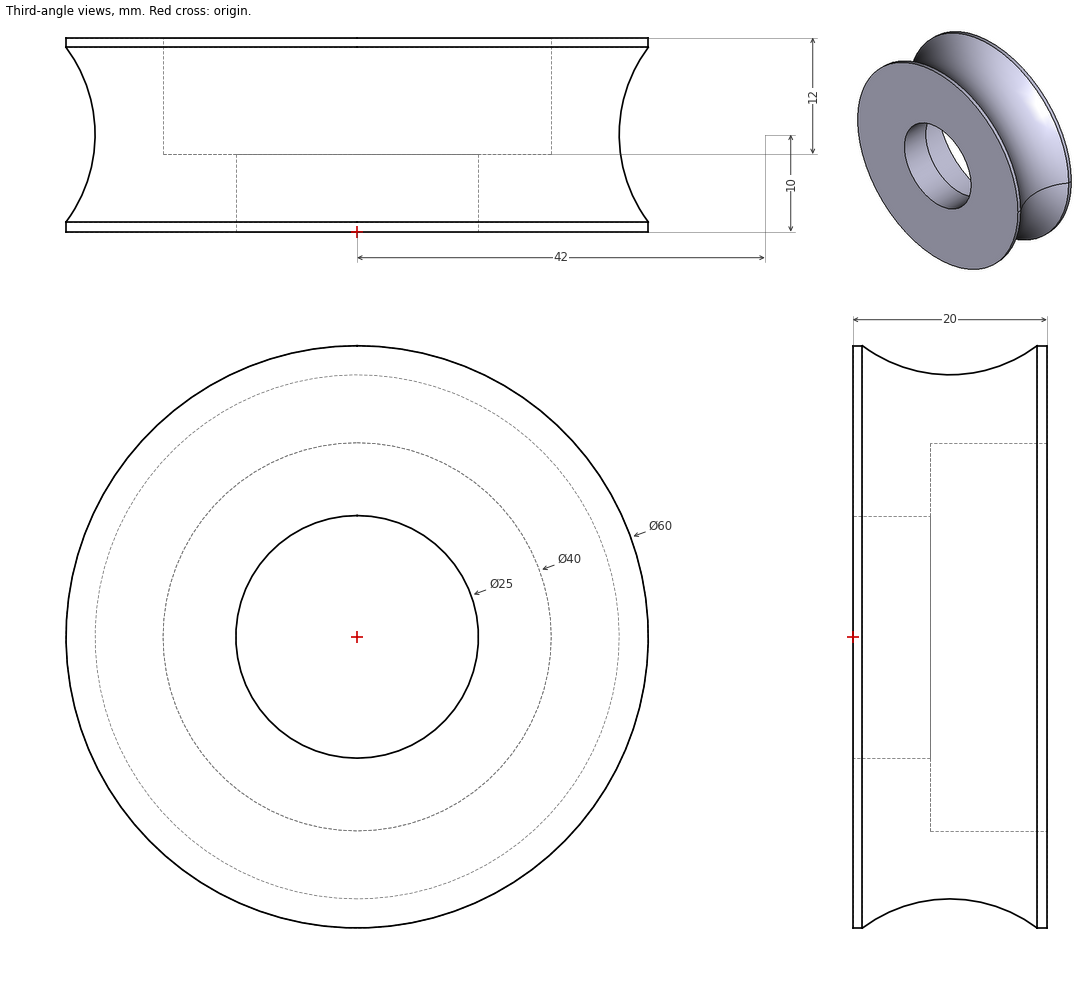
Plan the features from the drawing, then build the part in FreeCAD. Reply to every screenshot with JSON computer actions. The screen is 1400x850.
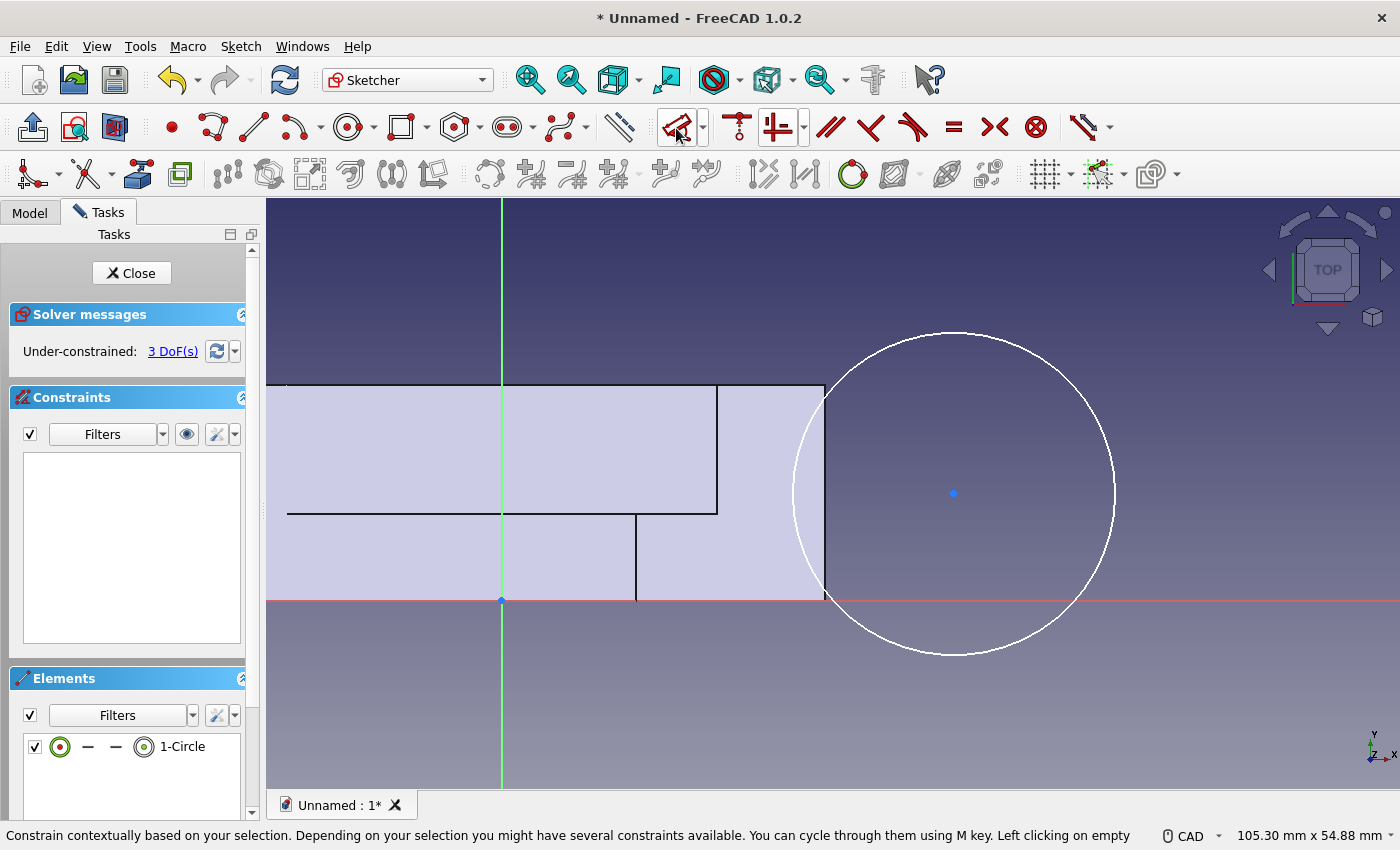
{"action": "left_click", "coordinate": [1068, 380]}
{"action": "left_click", "coordinate": [1091, 357]}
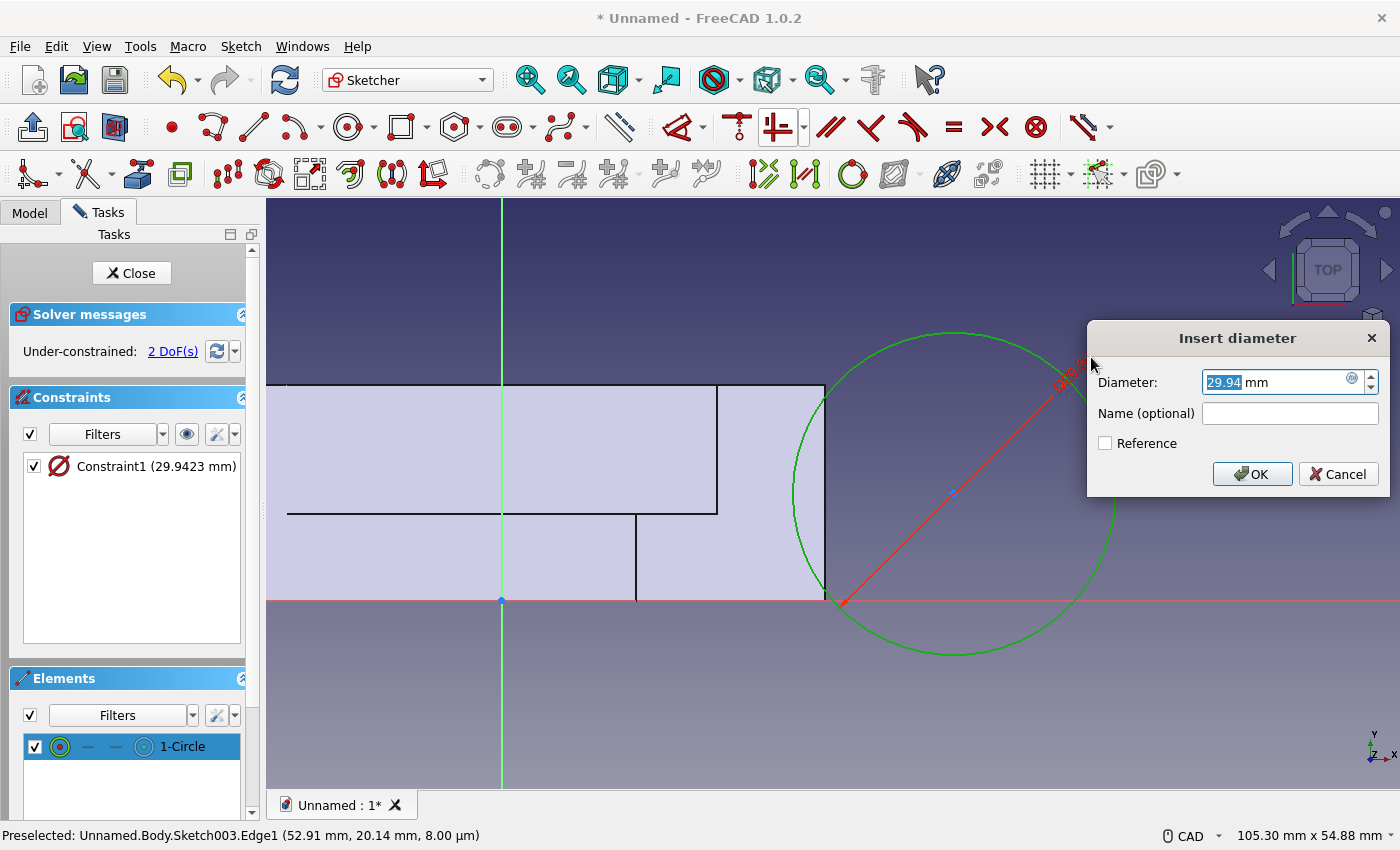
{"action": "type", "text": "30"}
{"action": "key", "text": "Return"}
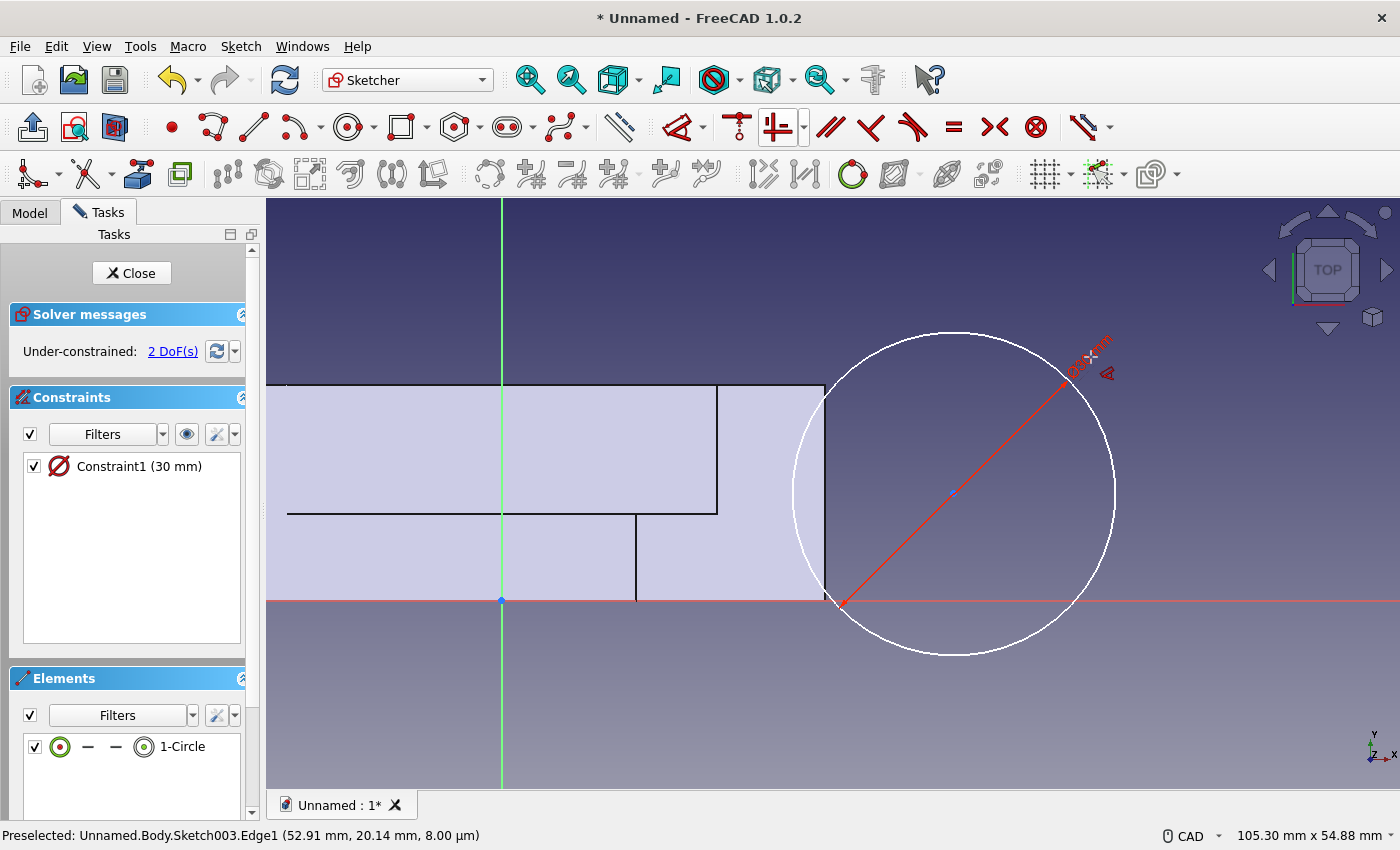
{"action": "left_click", "coordinate": [954, 494]}
{"action": "left_click", "coordinate": [728, 635]}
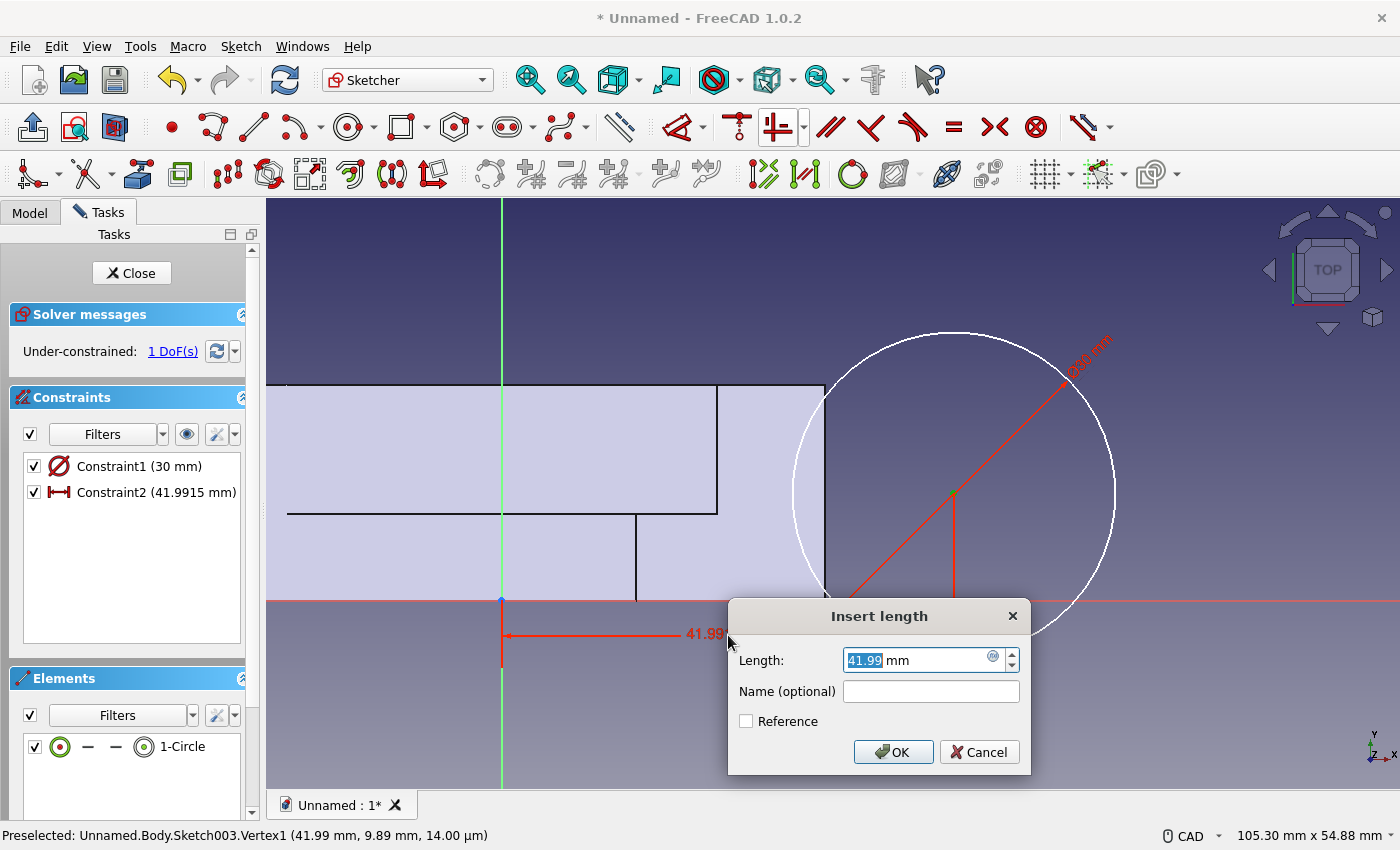
{"action": "type", "text": "42"}
{"action": "key", "text": "Return"}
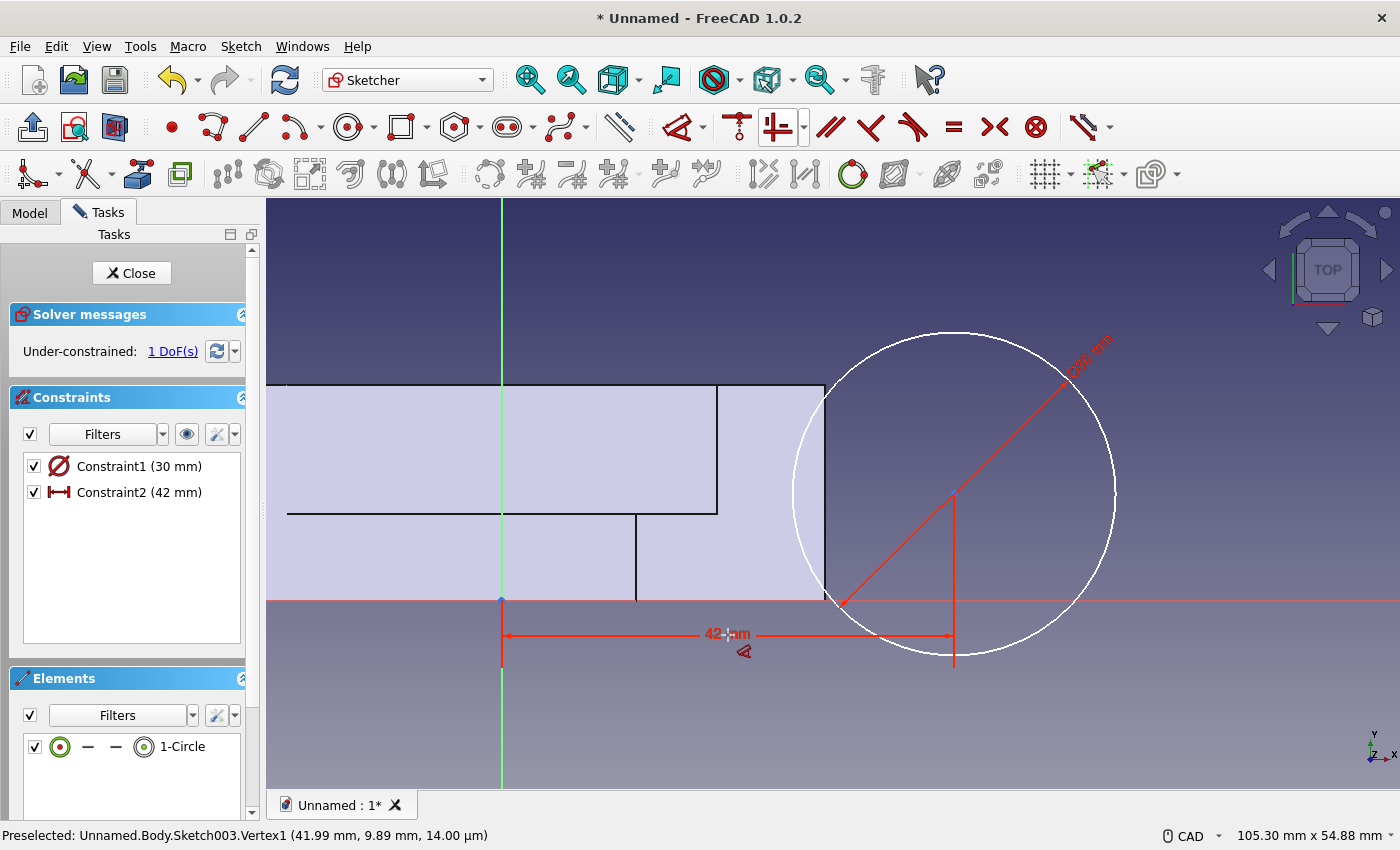
{"action": "left_click", "coordinate": [954, 494]}
{"action": "left_click", "coordinate": [468, 547]}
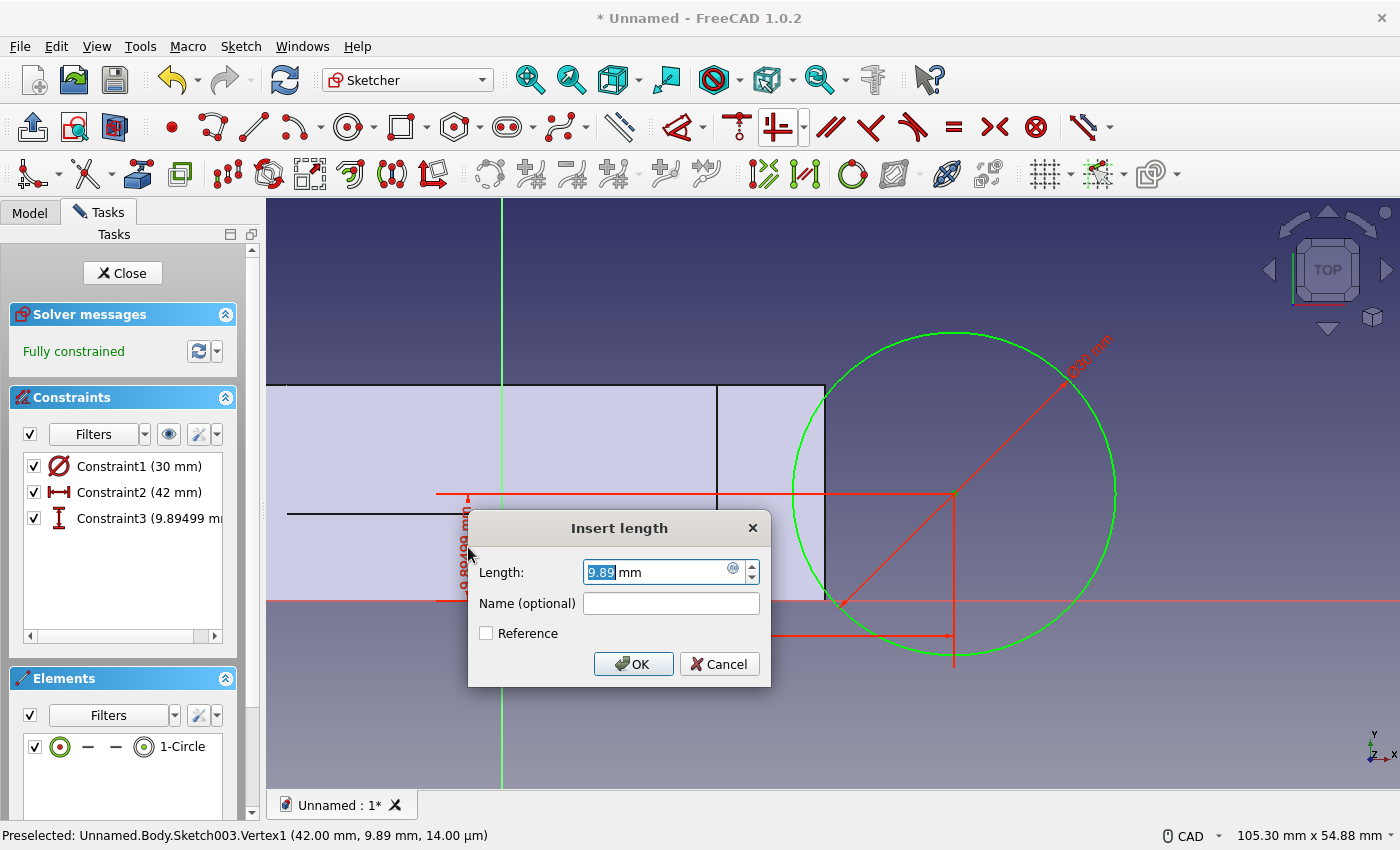
{"action": "type", "text": "10"}
{"action": "key", "text": "Return"}
{"action": "key", "text": "Escape"}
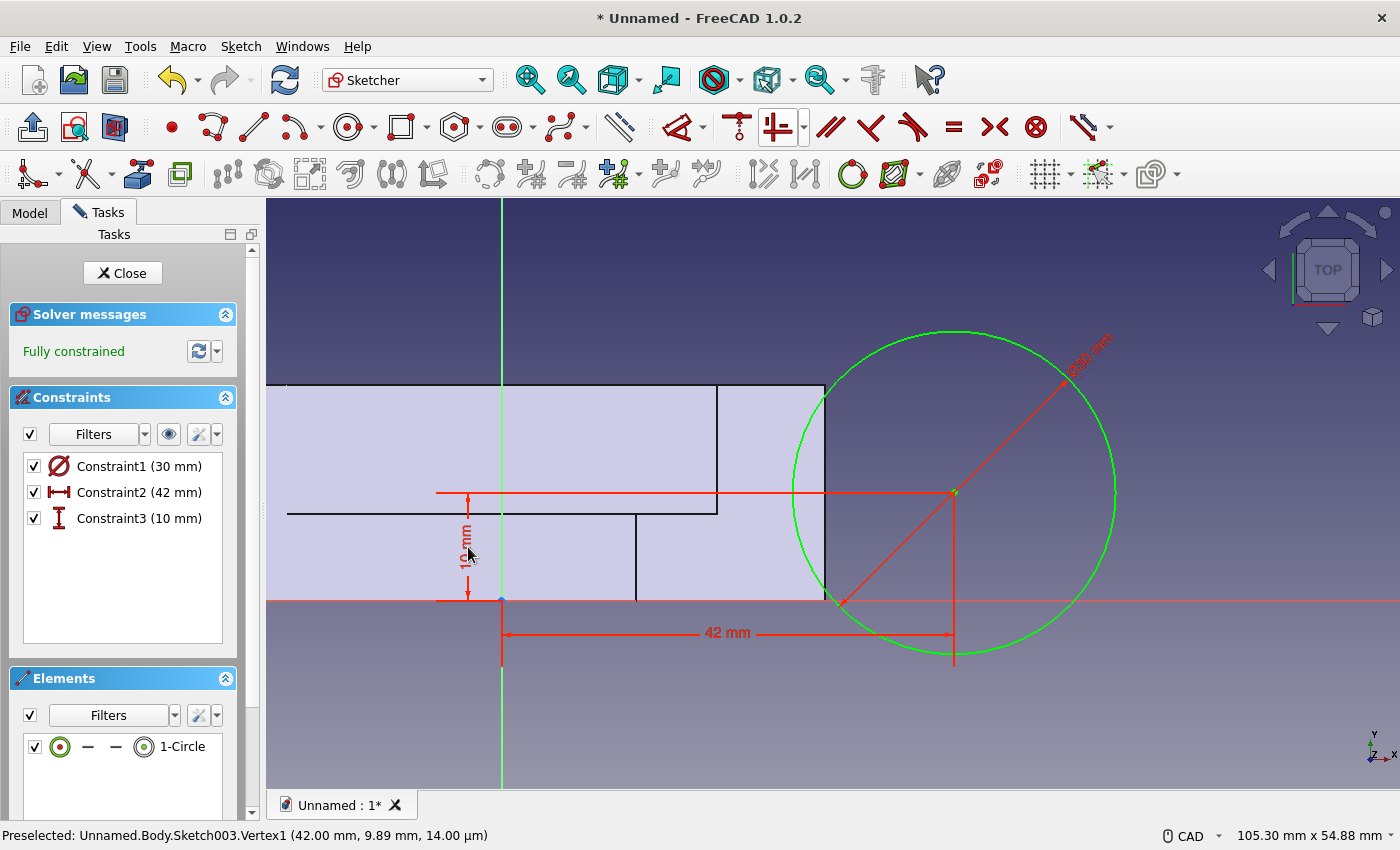
{"action": "left_click", "coordinate": [123, 273]}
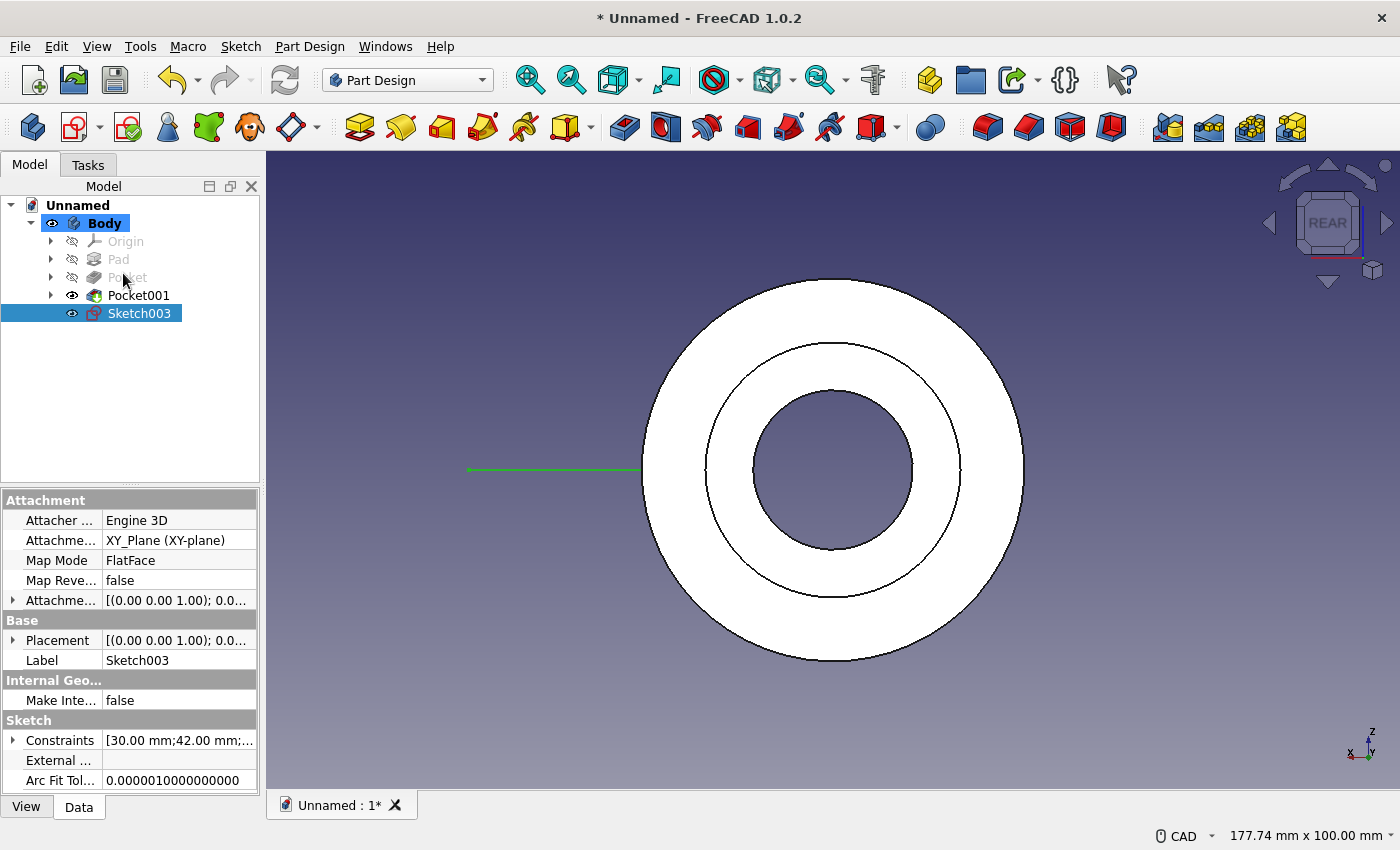
{"action": "left_click", "coordinate": [707, 128]}